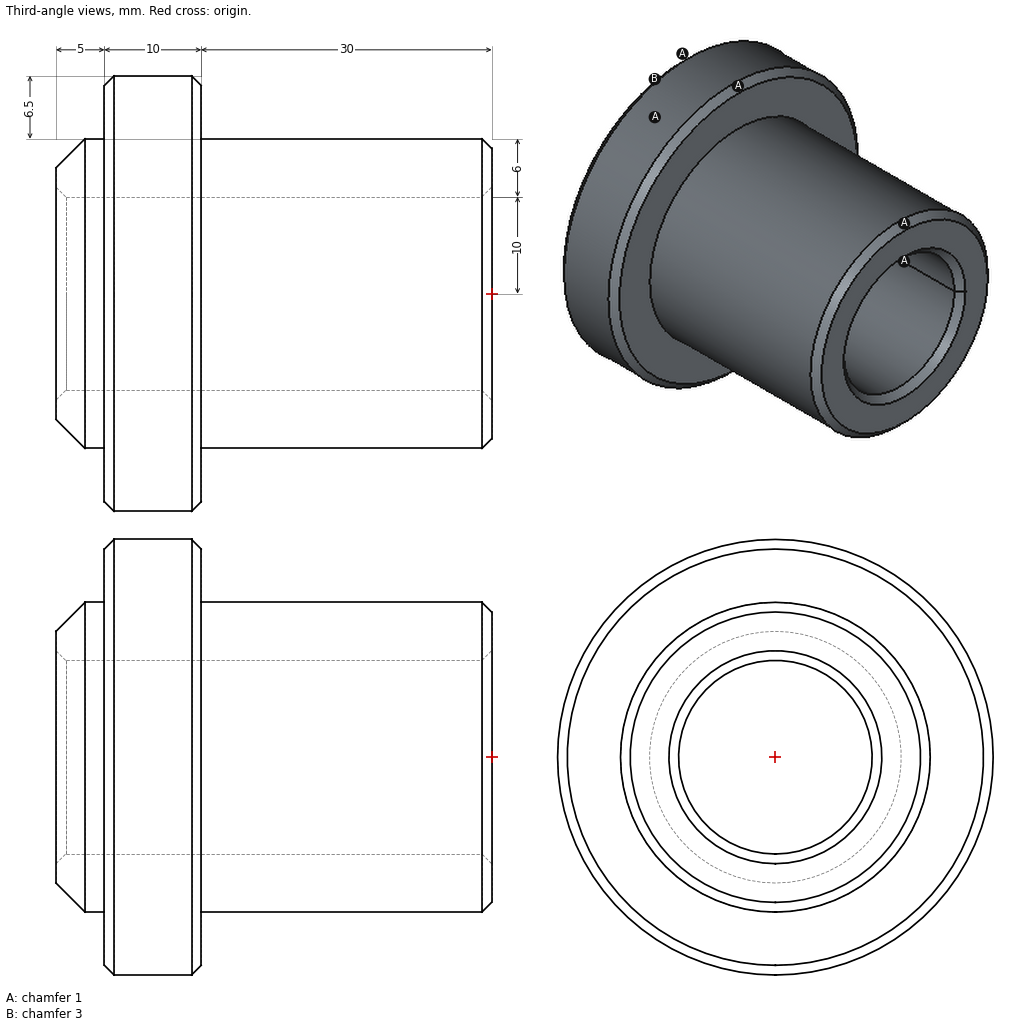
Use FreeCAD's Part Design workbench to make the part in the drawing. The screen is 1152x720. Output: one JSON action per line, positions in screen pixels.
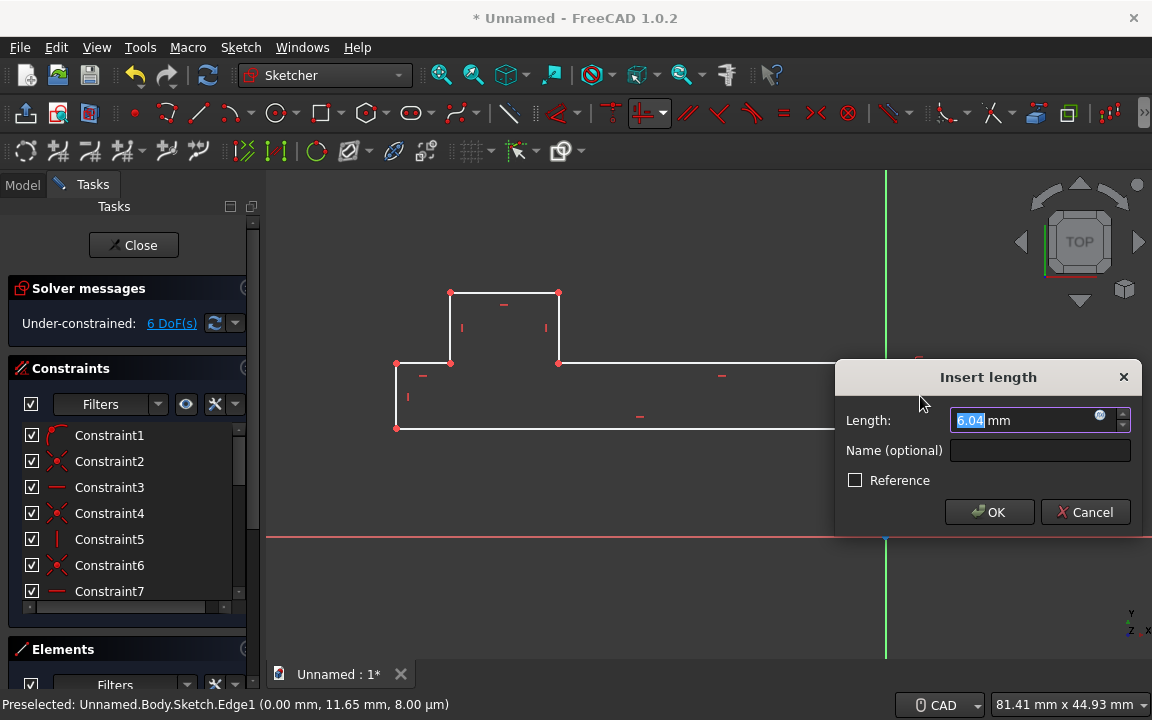
{"action": "type", "text": "6"}
{"action": "key", "text": "Return"}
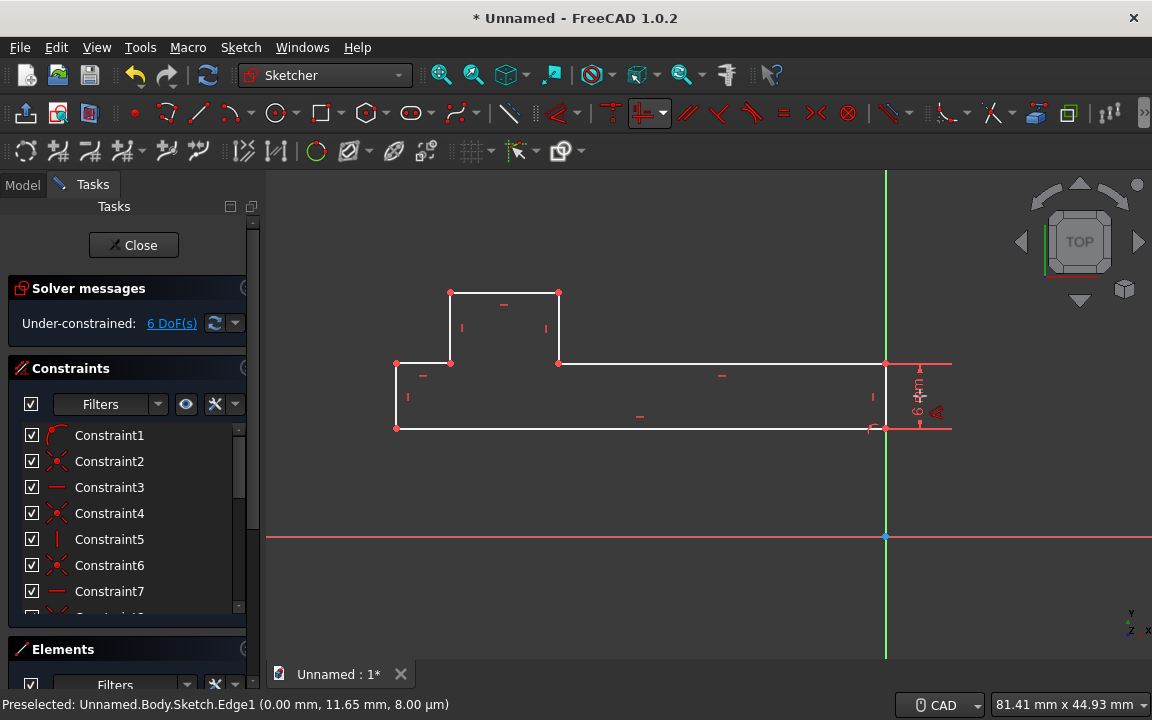
{"action": "left_click", "coordinate": [434, 363]}
{"action": "left_click", "coordinate": [423, 329]}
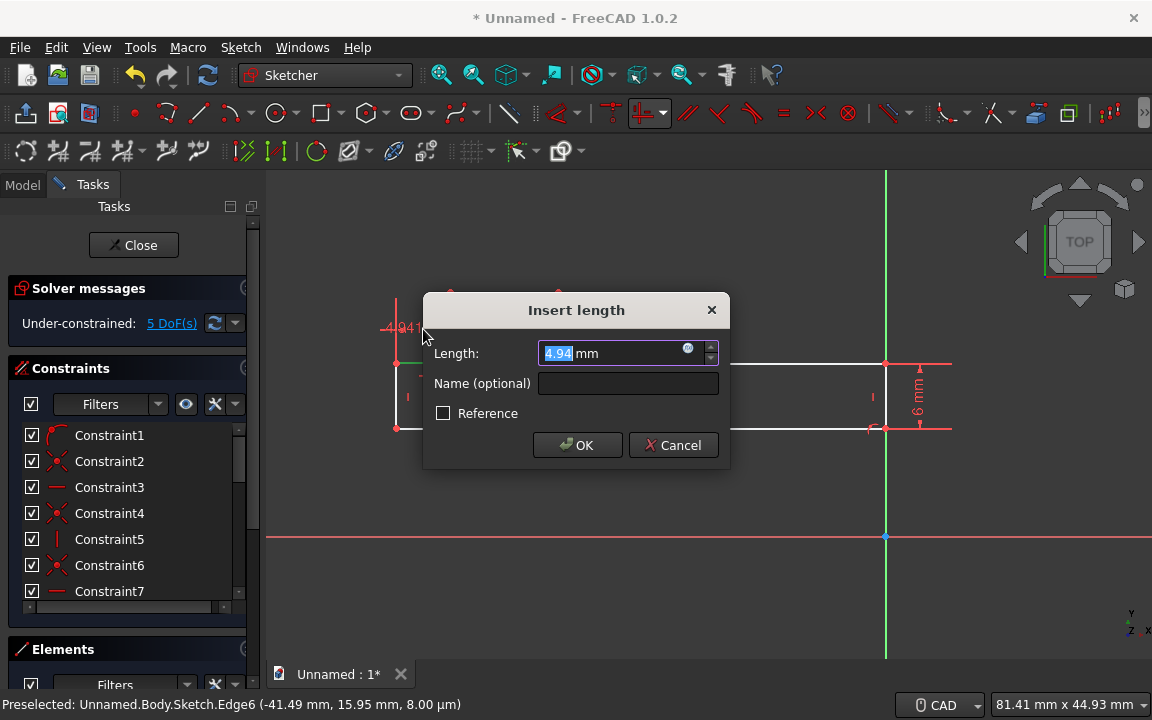
{"action": "type", "text": "5"}
{"action": "key", "text": "Return"}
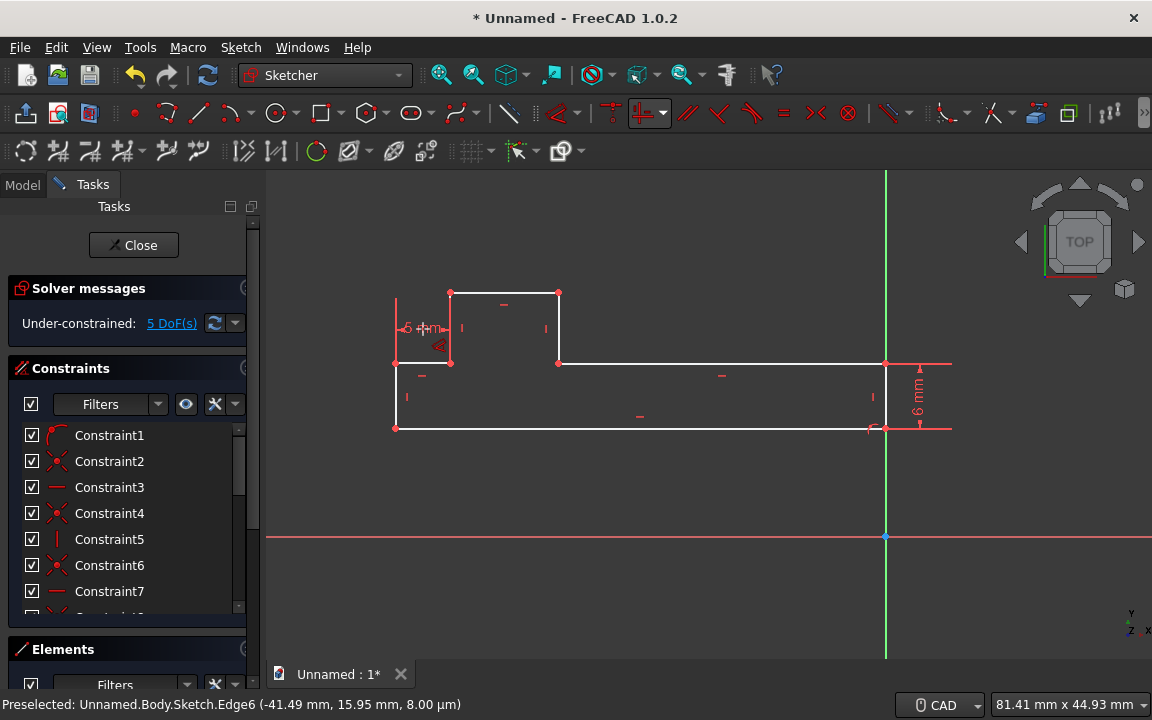
{"action": "left_click", "coordinate": [396, 383]}
{"action": "left_click", "coordinate": [362, 396]}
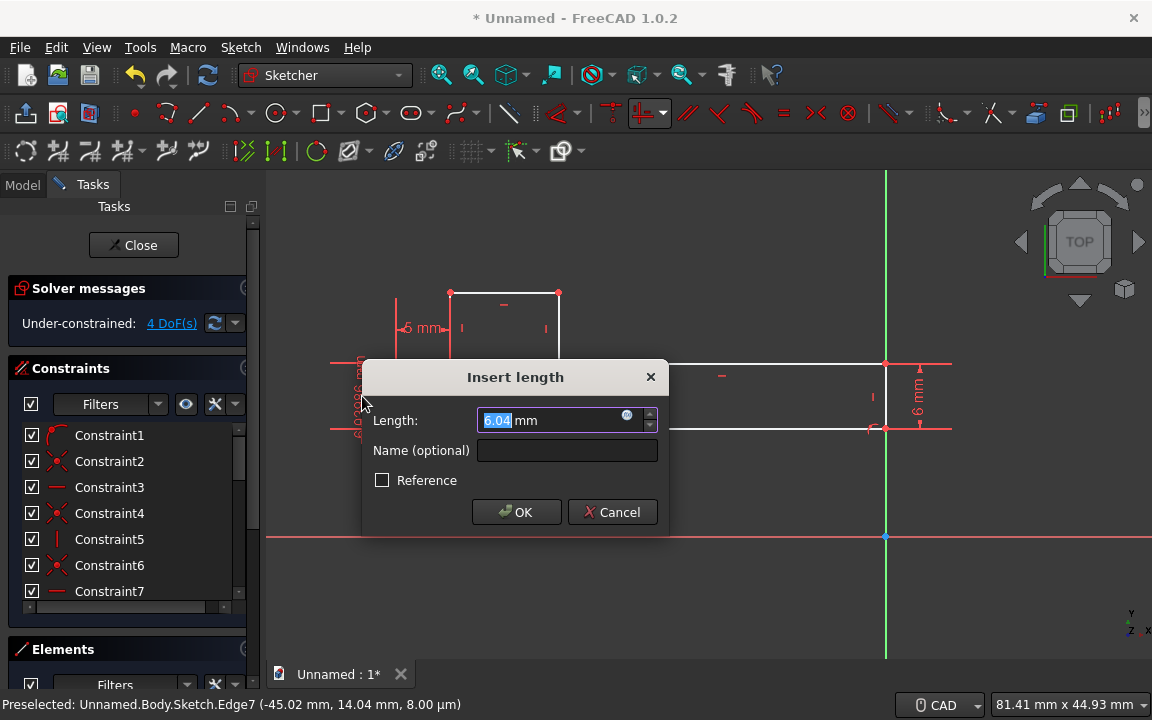
{"action": "type", "text": "6"}
{"action": "key", "text": "Return"}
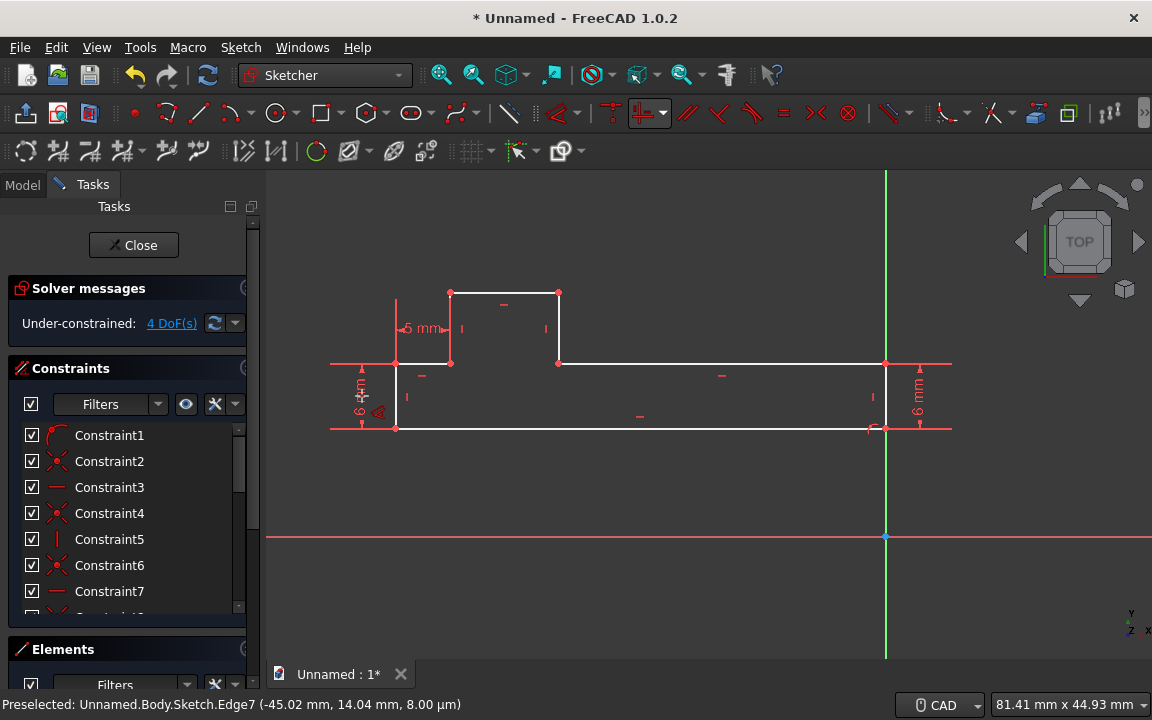
{"action": "left_click", "coordinate": [787, 364]}
{"action": "left_click", "coordinate": [722, 330]}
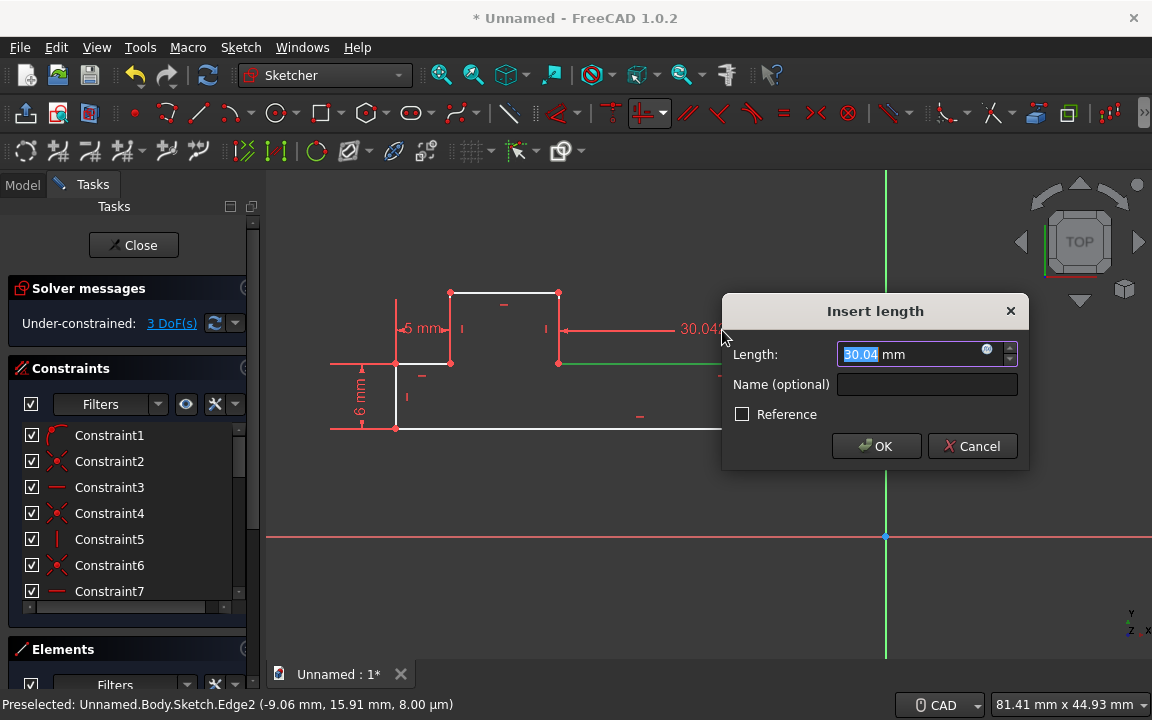
{"action": "type", "text": "30"}
{"action": "key", "text": "Return"}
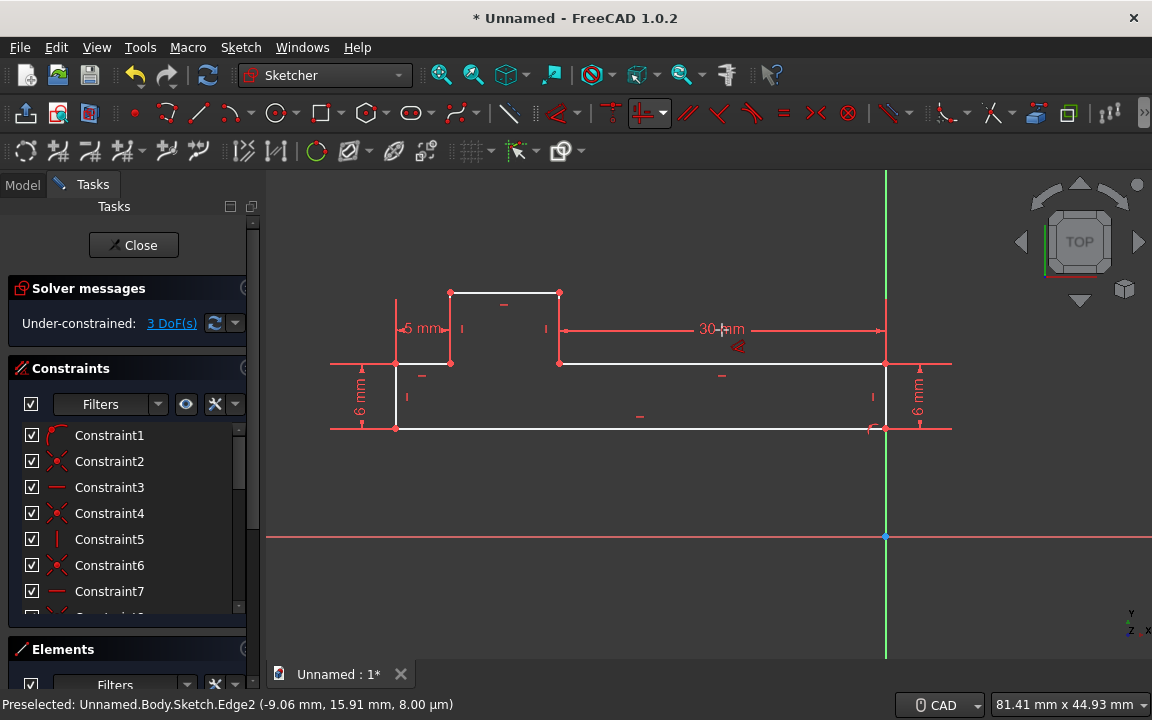
{"action": "left_click", "coordinate": [526, 292]}
{"action": "left_click", "coordinate": [505, 258]}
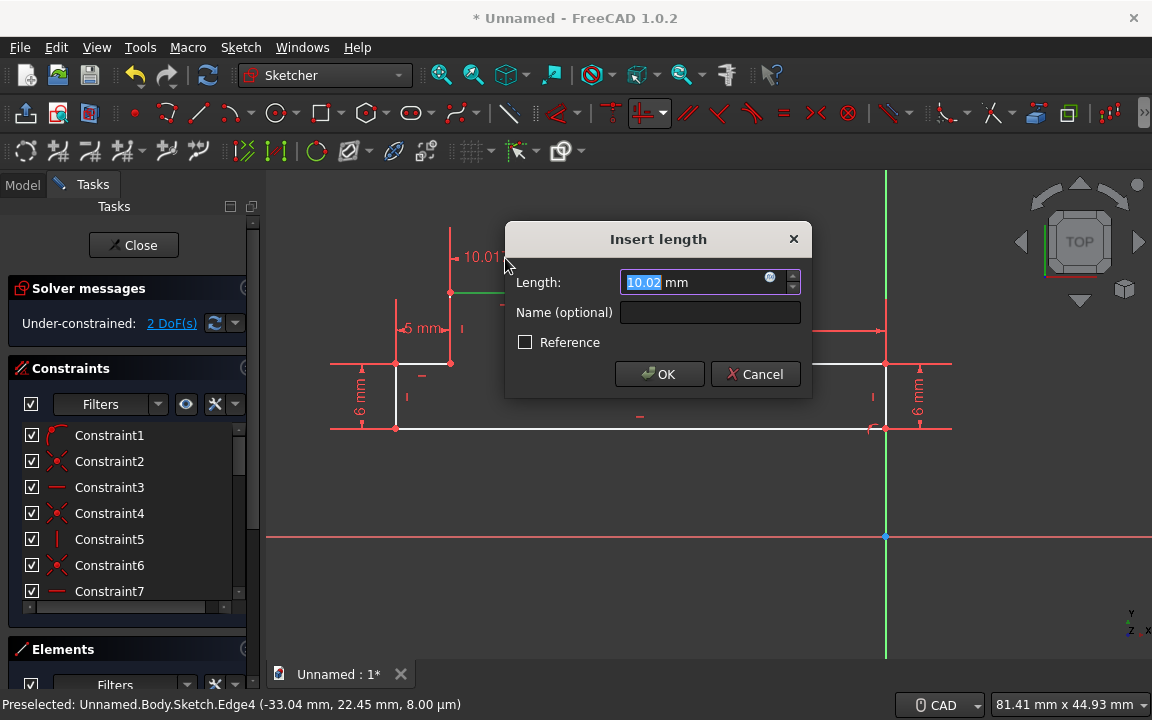
{"action": "type", "text": "10"}
{"action": "key", "text": "Return"}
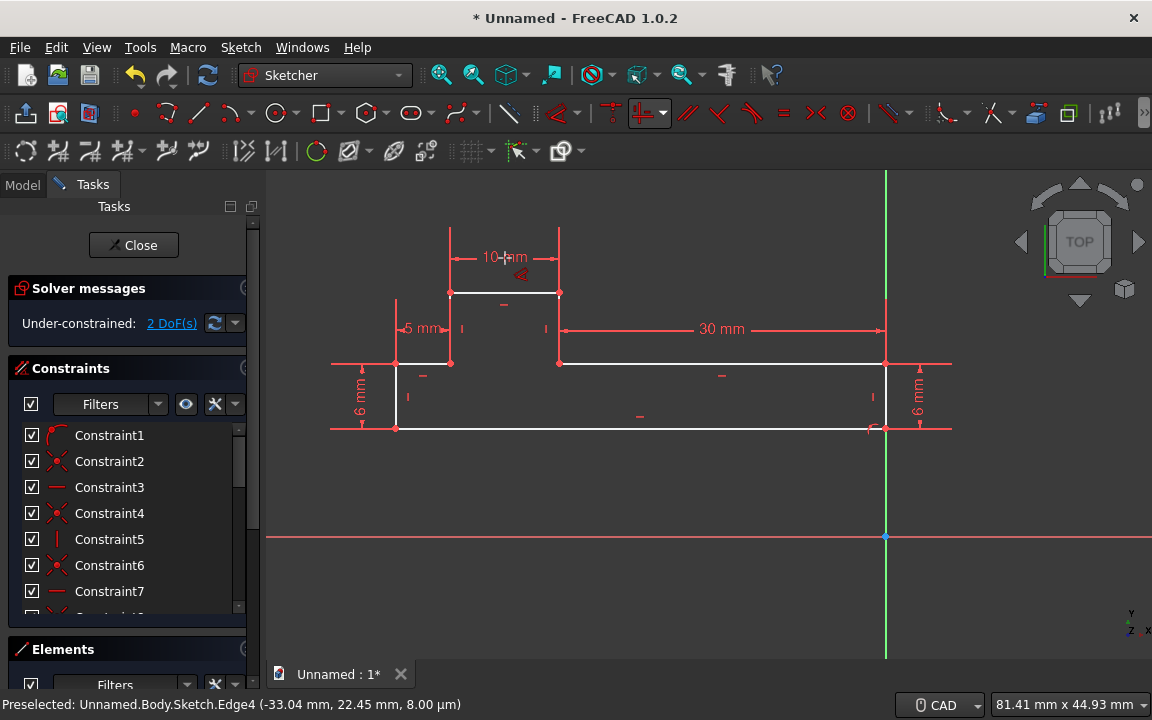
{"action": "left_click", "coordinate": [559, 342]}
{"action": "left_click", "coordinate": [525, 328]}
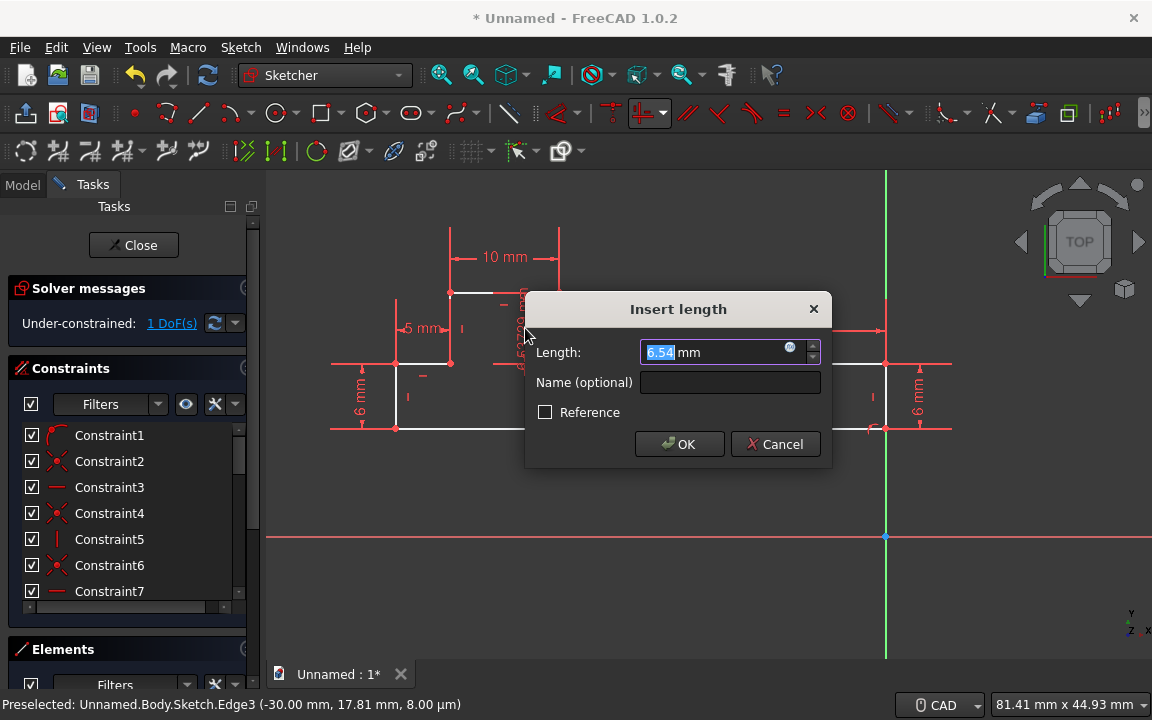
{"action": "type", "text": "6.5"}
{"action": "key", "text": "Return"}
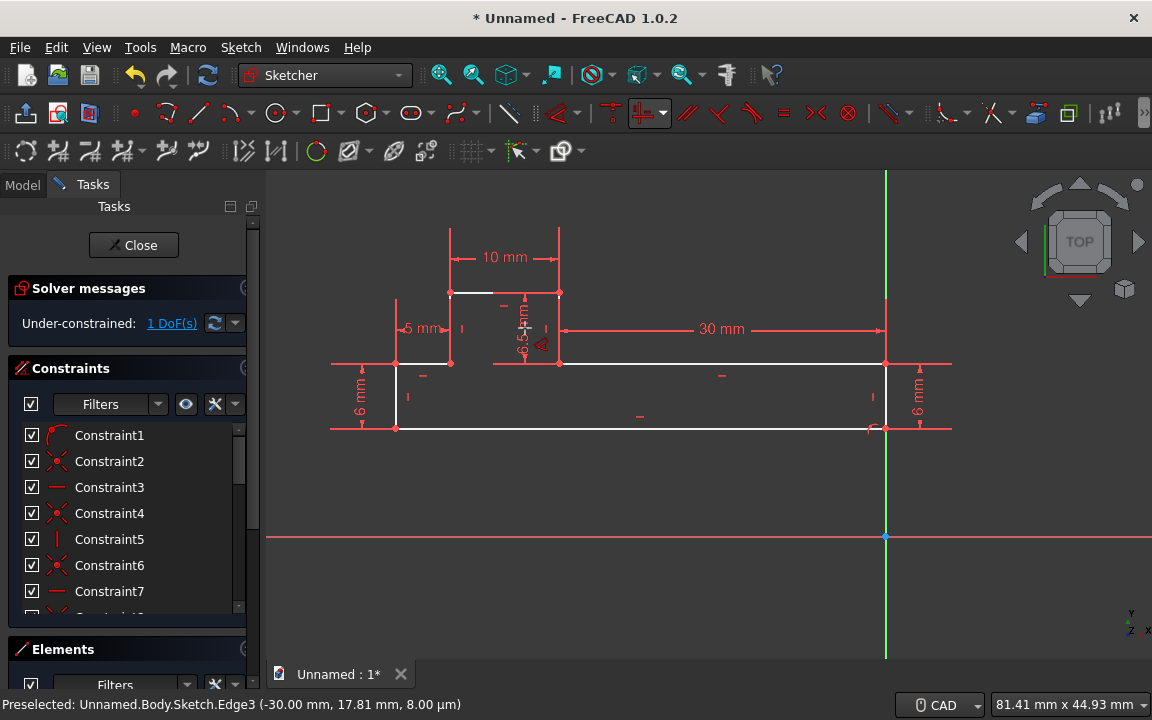
{"action": "left_click", "coordinate": [886, 429]}
{"action": "left_click", "coordinate": [920, 483]}